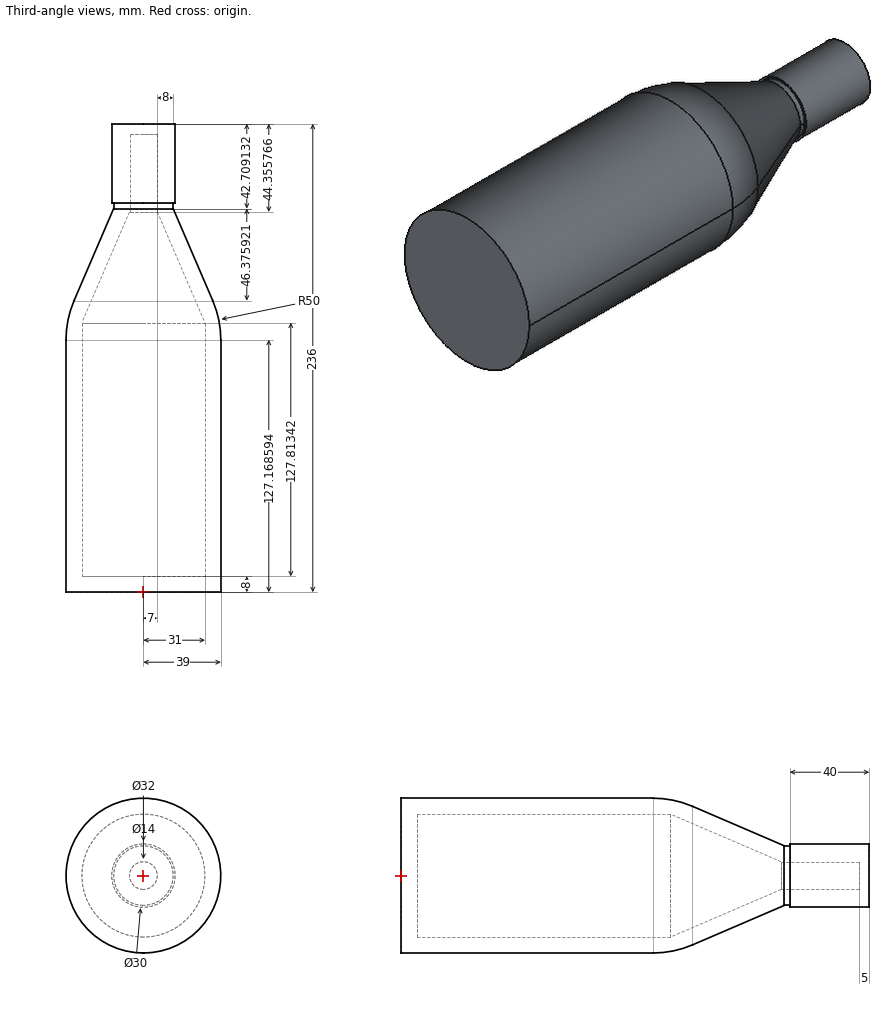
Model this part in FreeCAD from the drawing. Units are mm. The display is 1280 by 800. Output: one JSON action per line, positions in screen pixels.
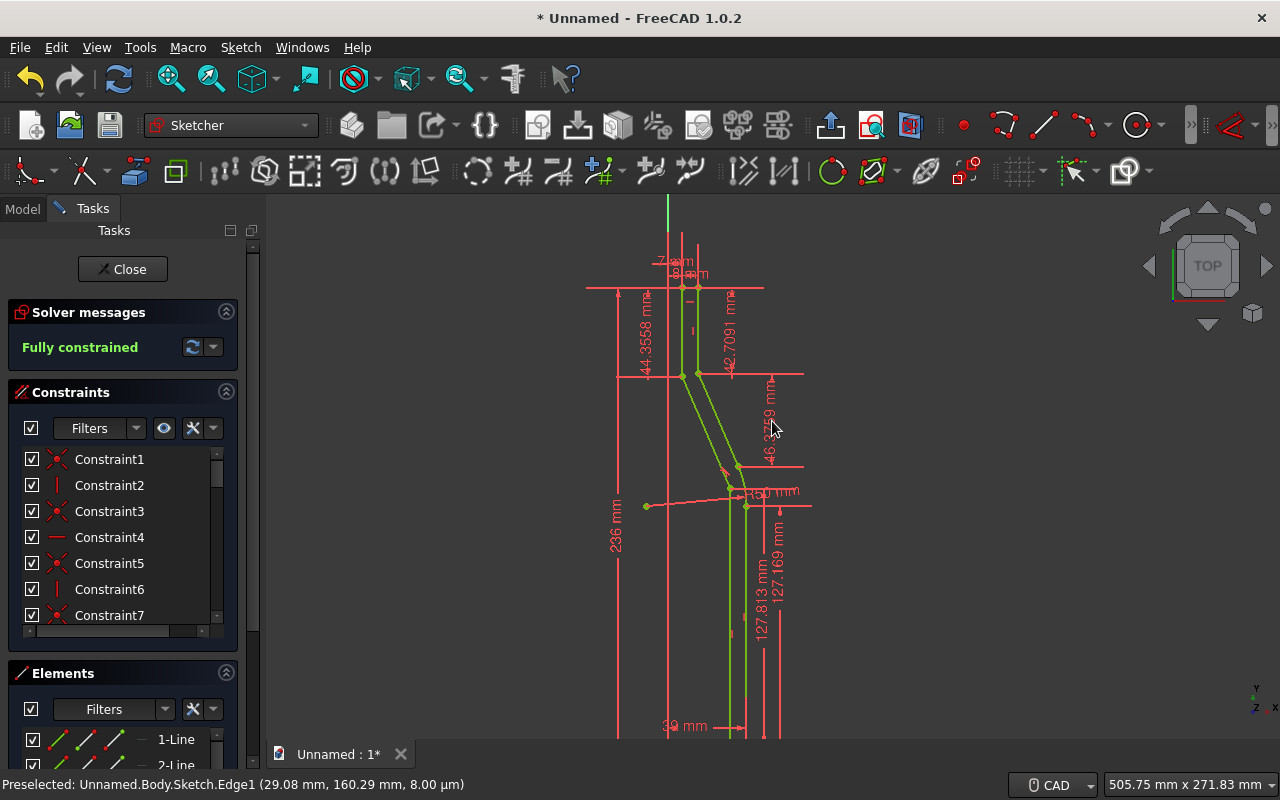
{"action": "left_click", "coordinate": [123, 269]}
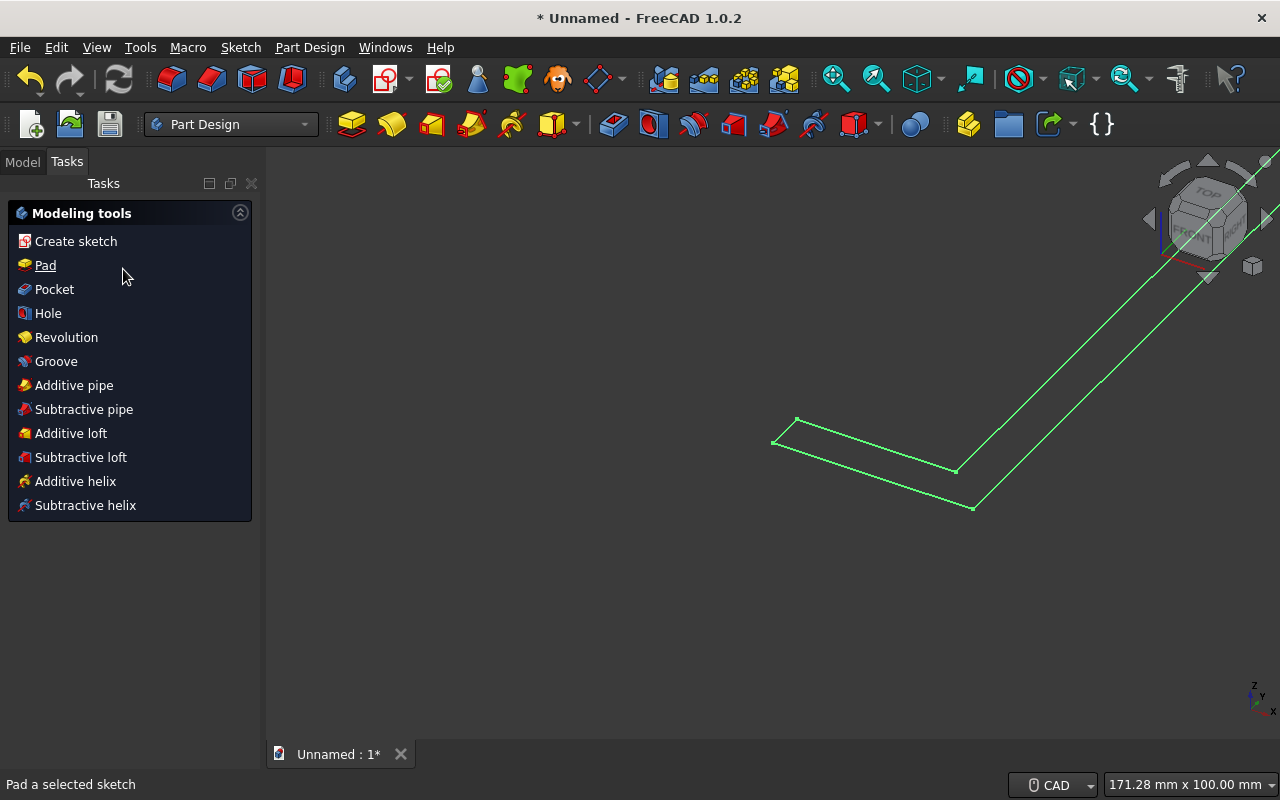
{"action": "left_click", "coordinate": [392, 124]}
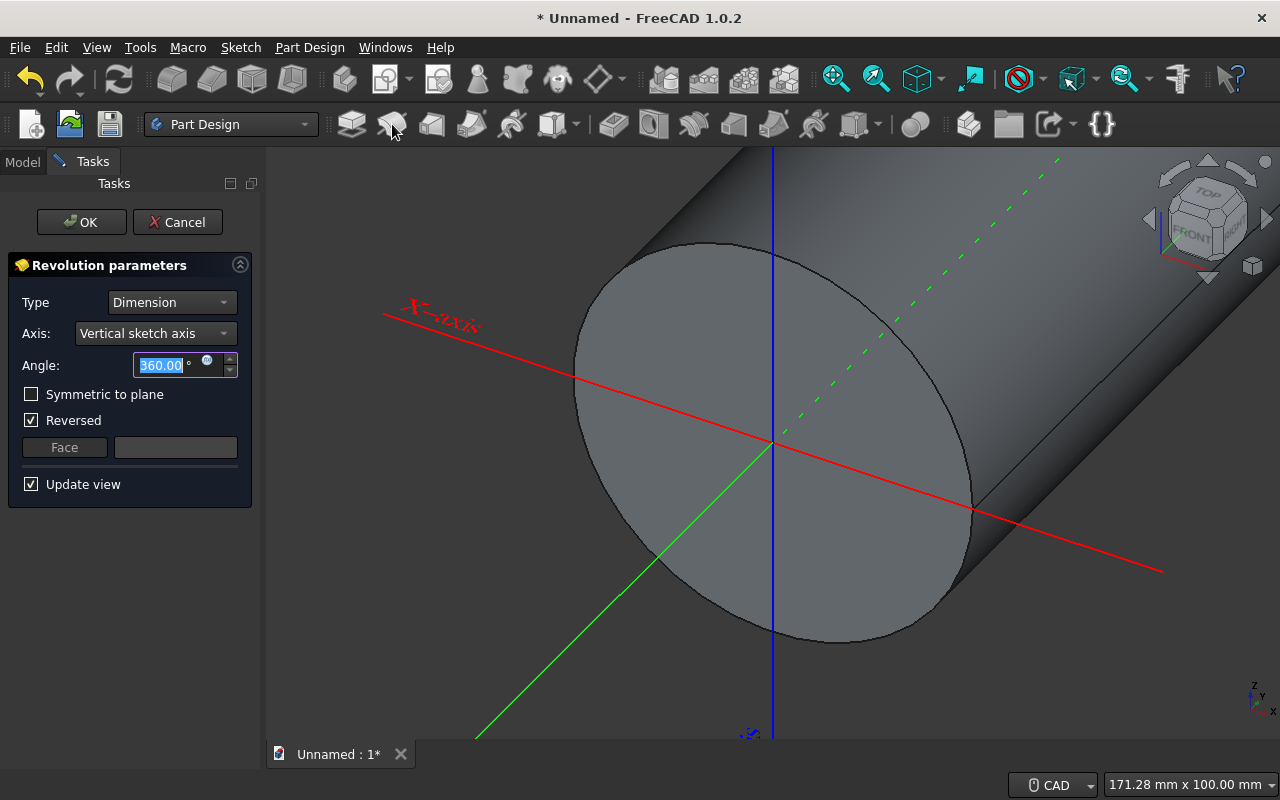
{"action": "left_click", "coordinate": [82, 222]}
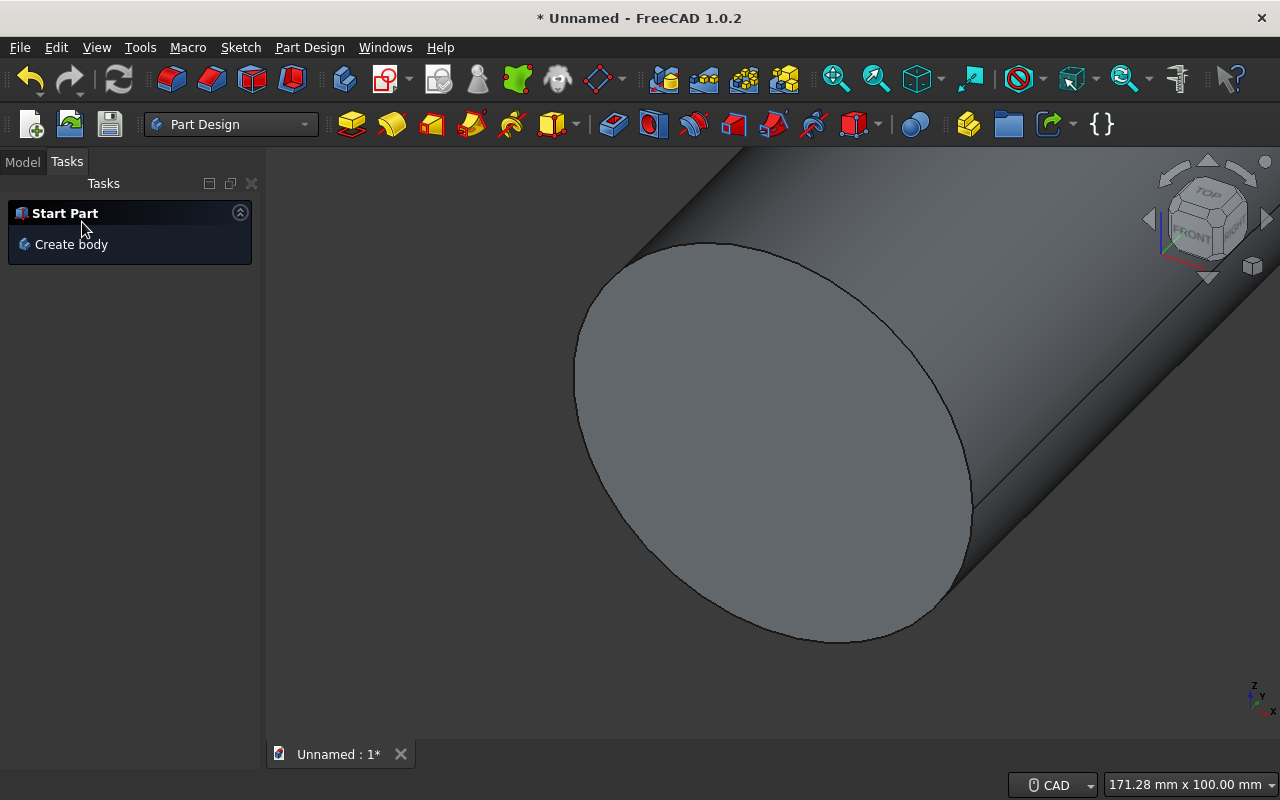
{"action": "key", "text": "v f"}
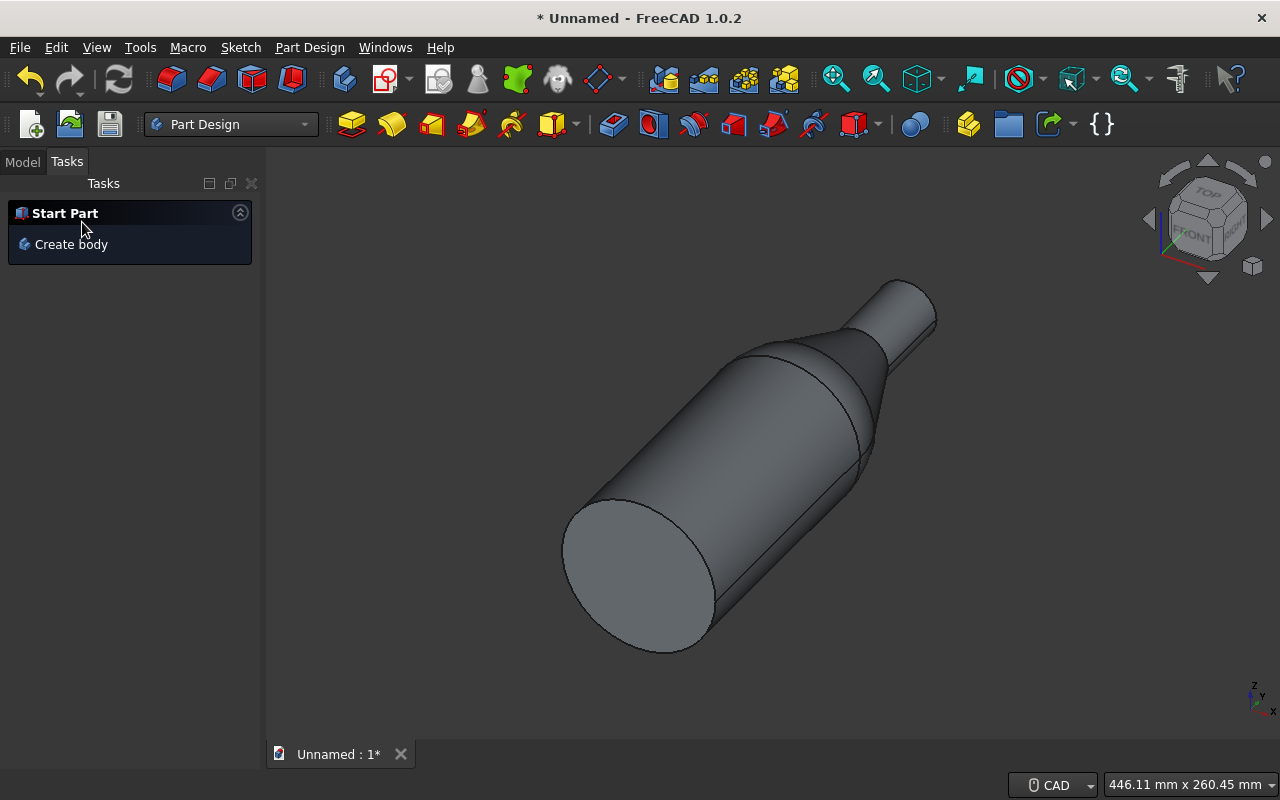
{"action": "left_click", "coordinate": [23, 161]}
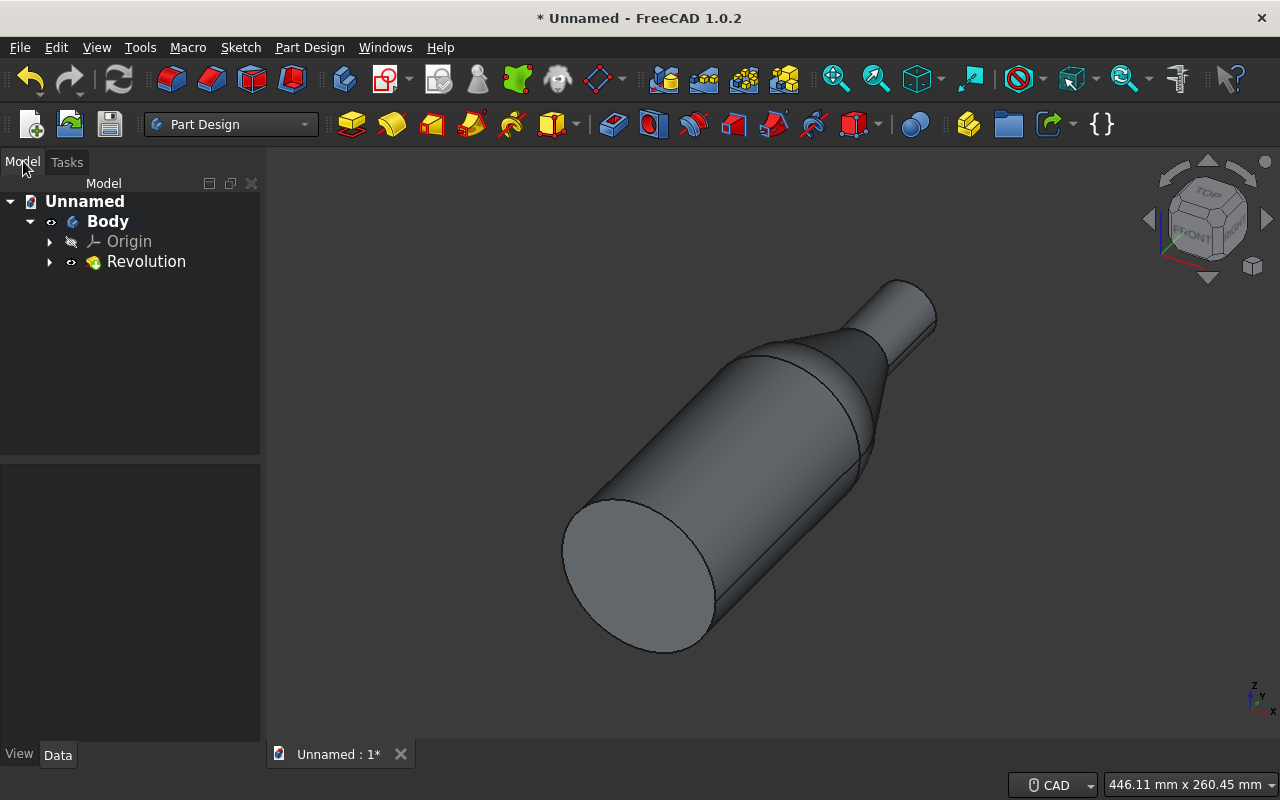
{"action": "left_click", "coordinate": [50, 242]}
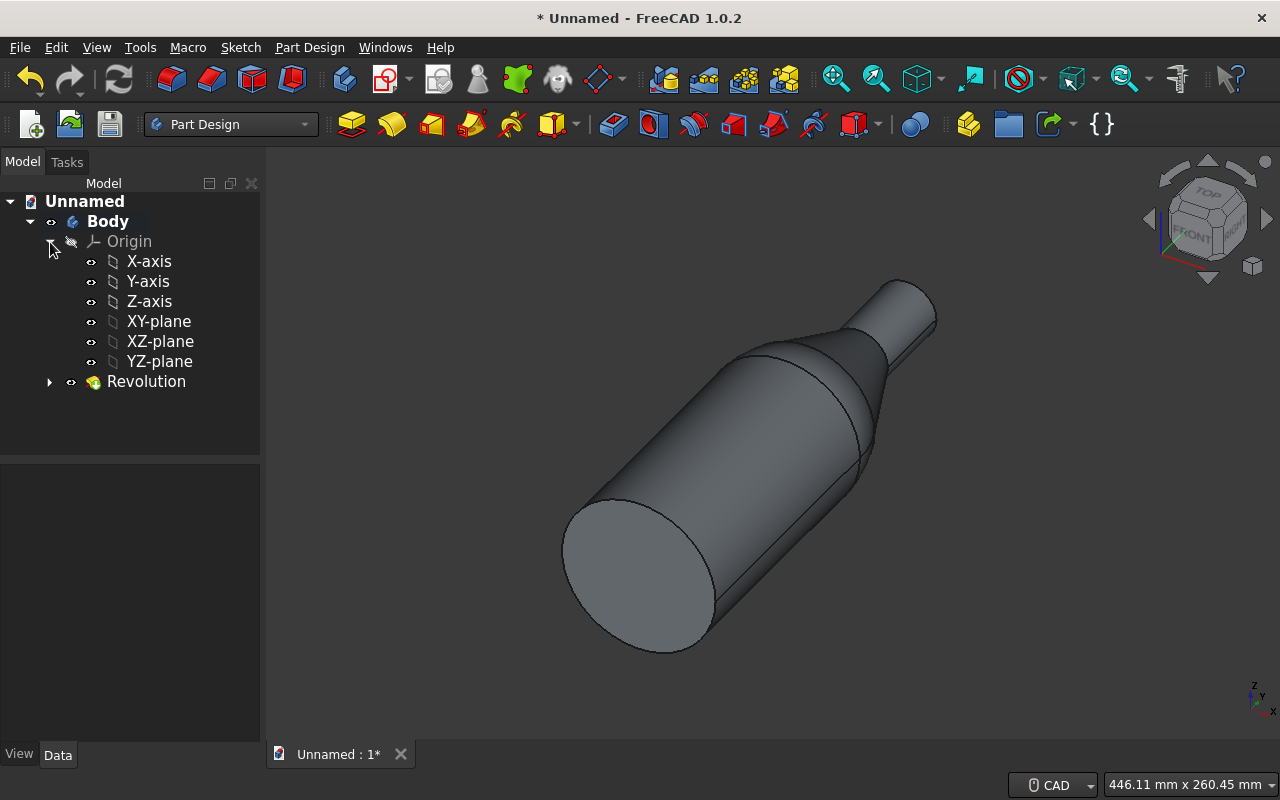
{"action": "left_click", "coordinate": [136, 342]}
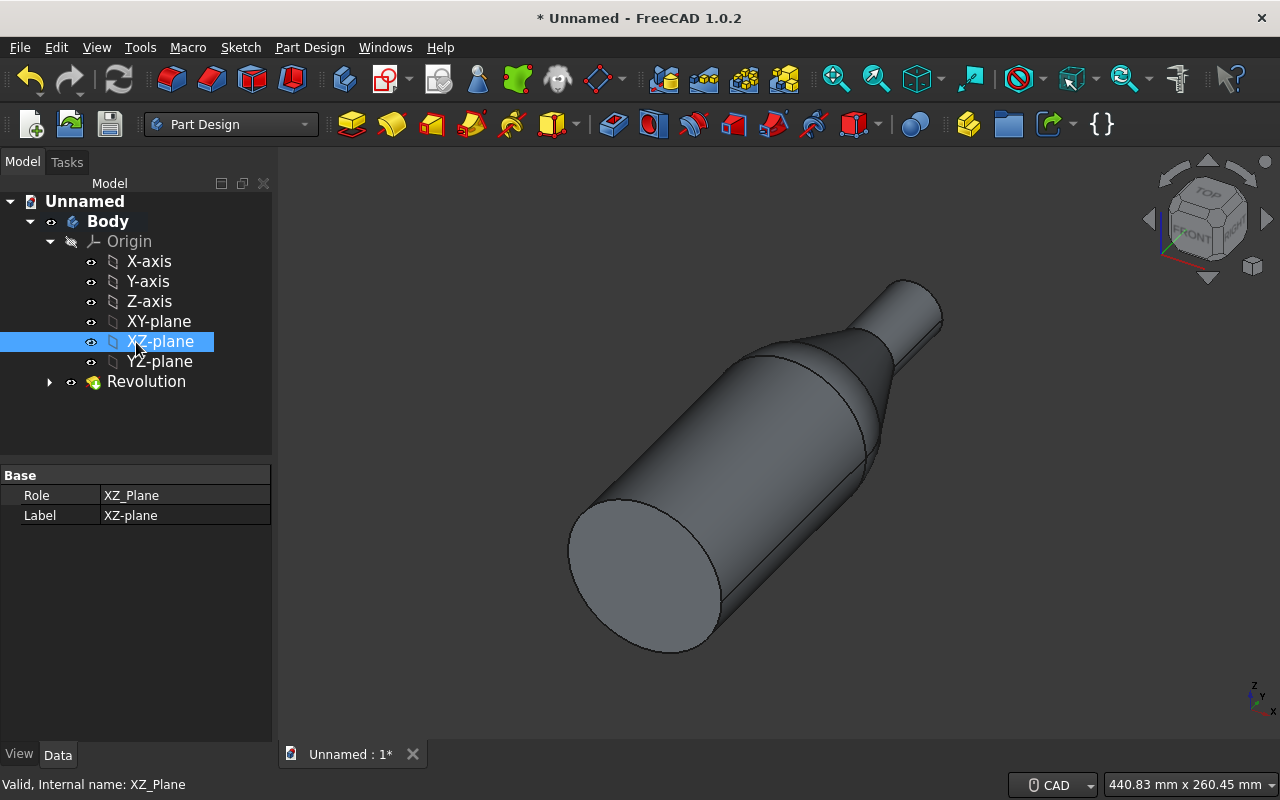
{"action": "left_click", "coordinate": [598, 80]}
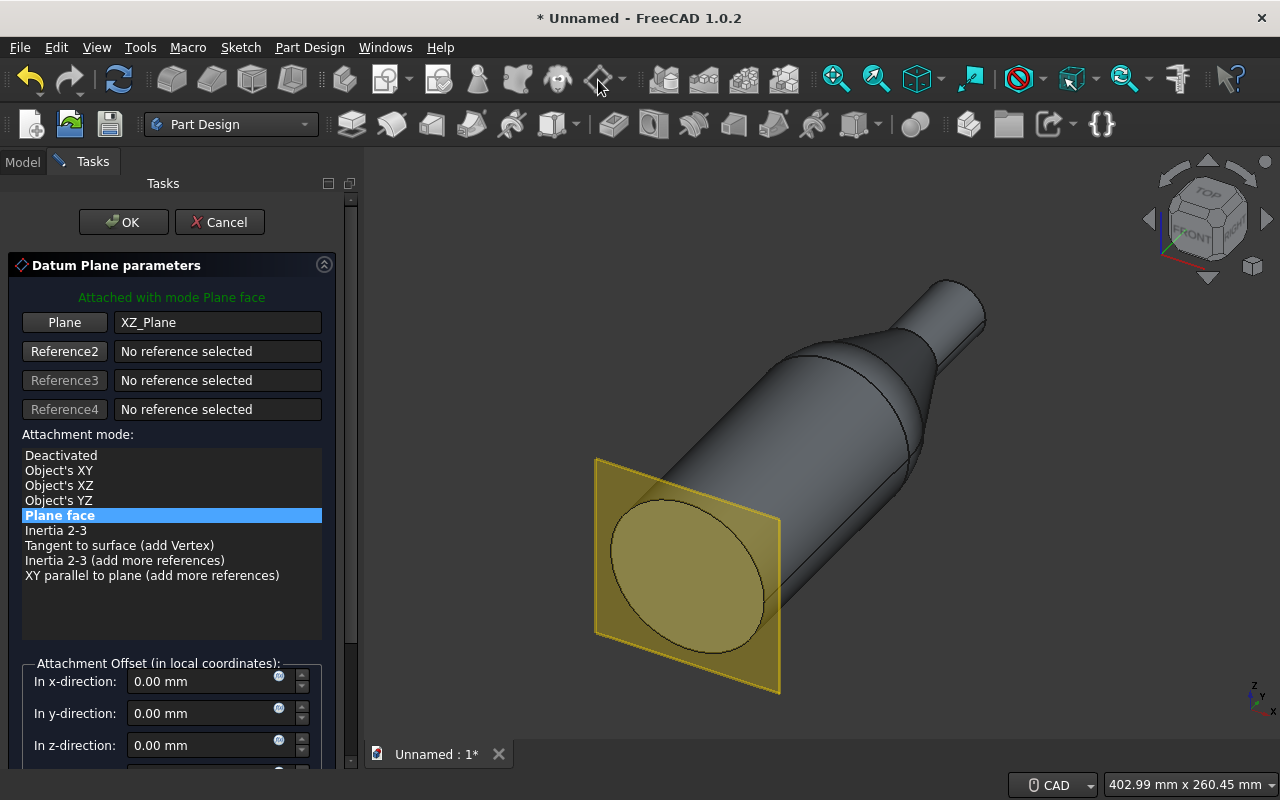
{"action": "triple_click", "coordinate": [210, 745]}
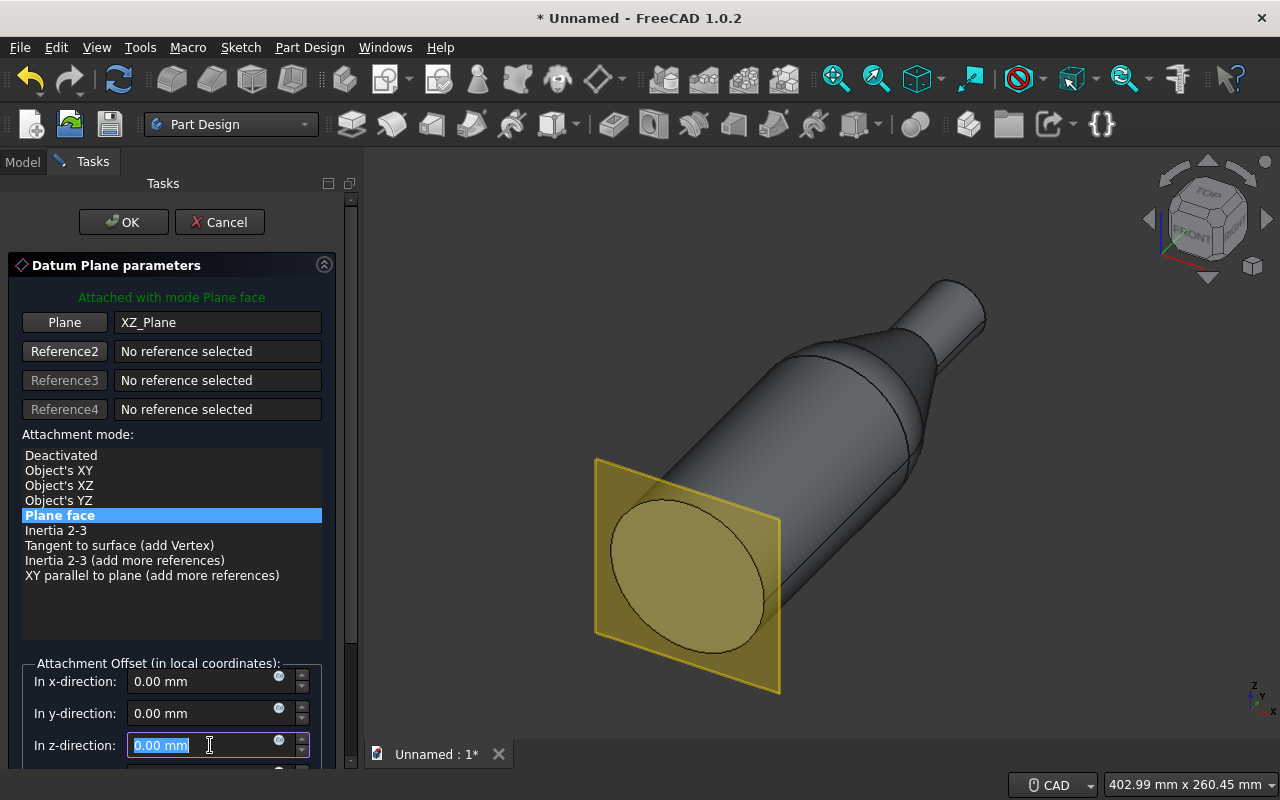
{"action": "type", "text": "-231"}
{"action": "key", "text": "Tab"}